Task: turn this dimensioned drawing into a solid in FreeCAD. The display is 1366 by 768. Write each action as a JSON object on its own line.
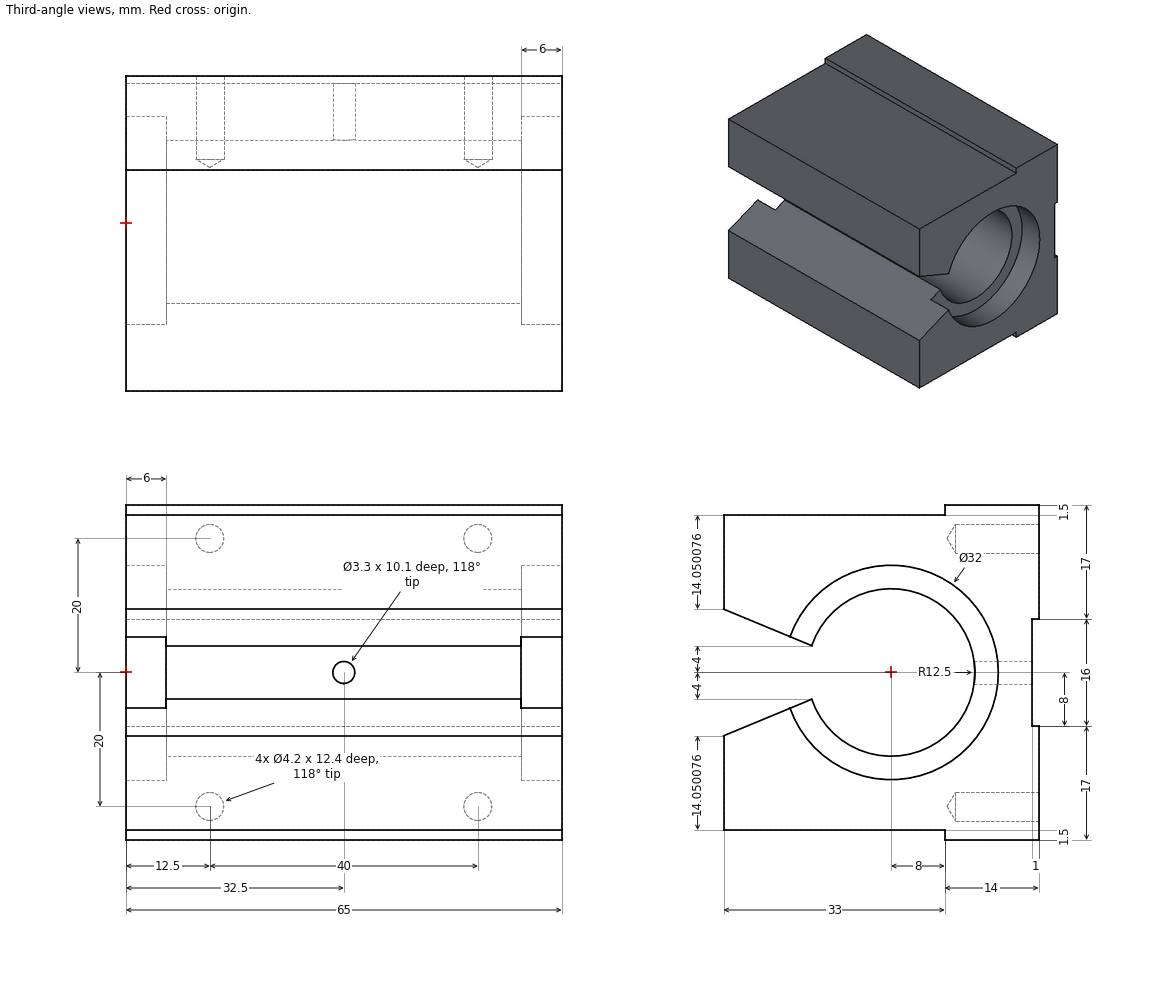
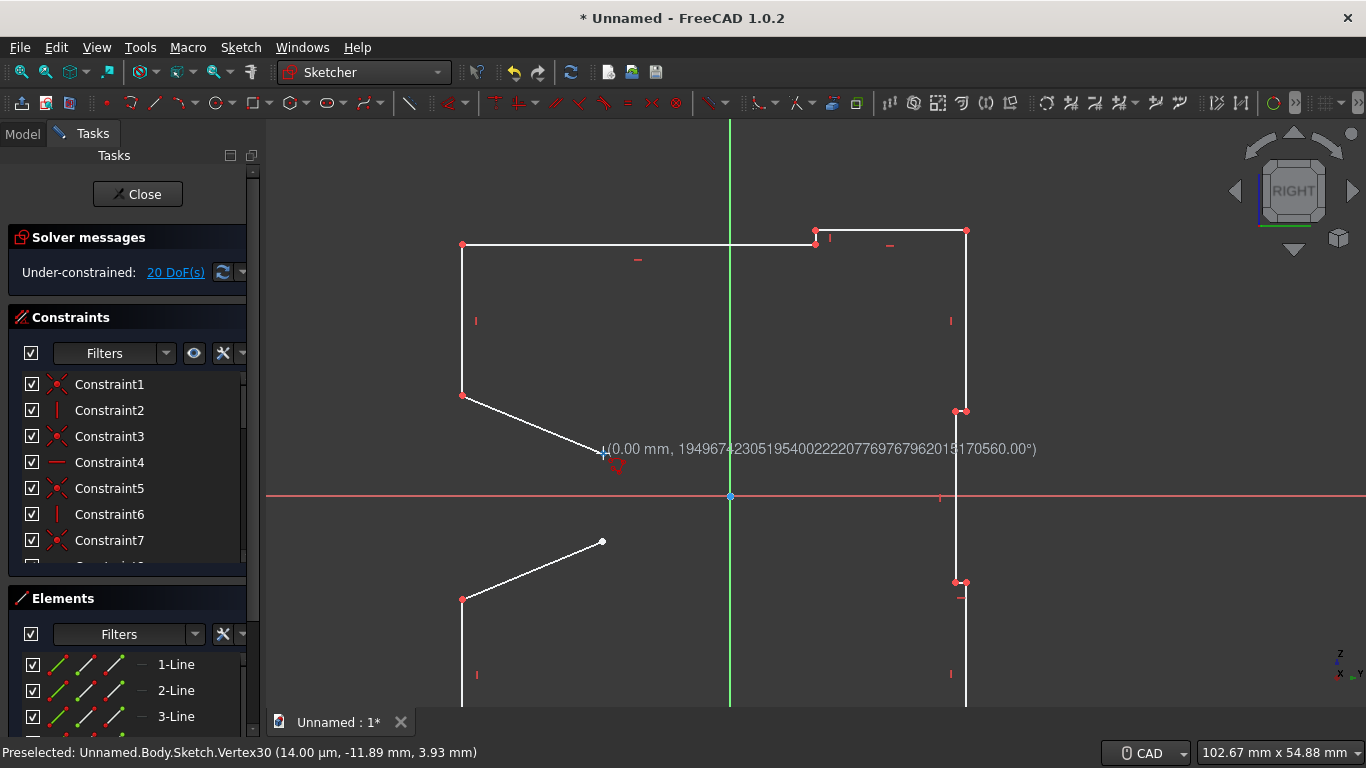
{"action": "key", "text": "g 3 a"}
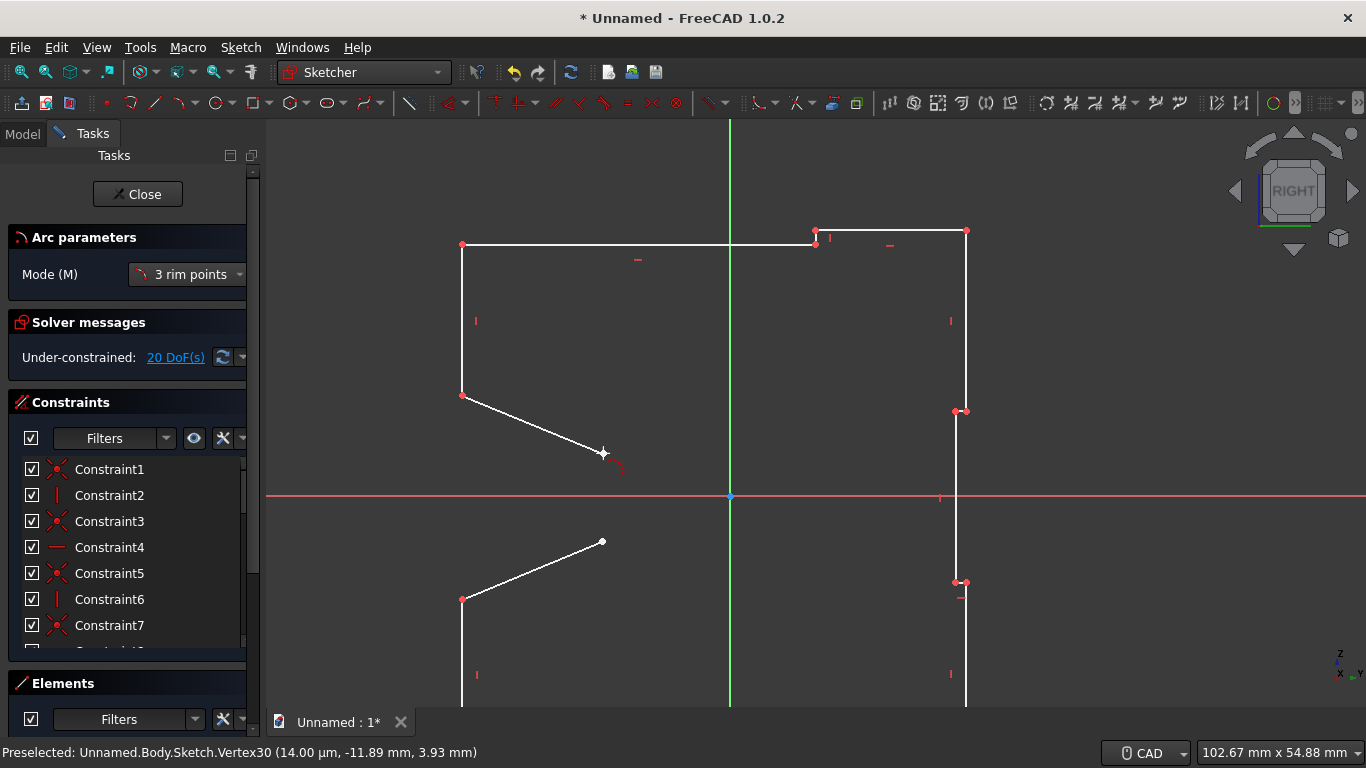
{"action": "left_click", "coordinate": [603, 454]}
{"action": "left_click", "coordinate": [603, 542]}
{"action": "left_click", "coordinate": [844, 568]}
{"action": "key", "text": "Escape"}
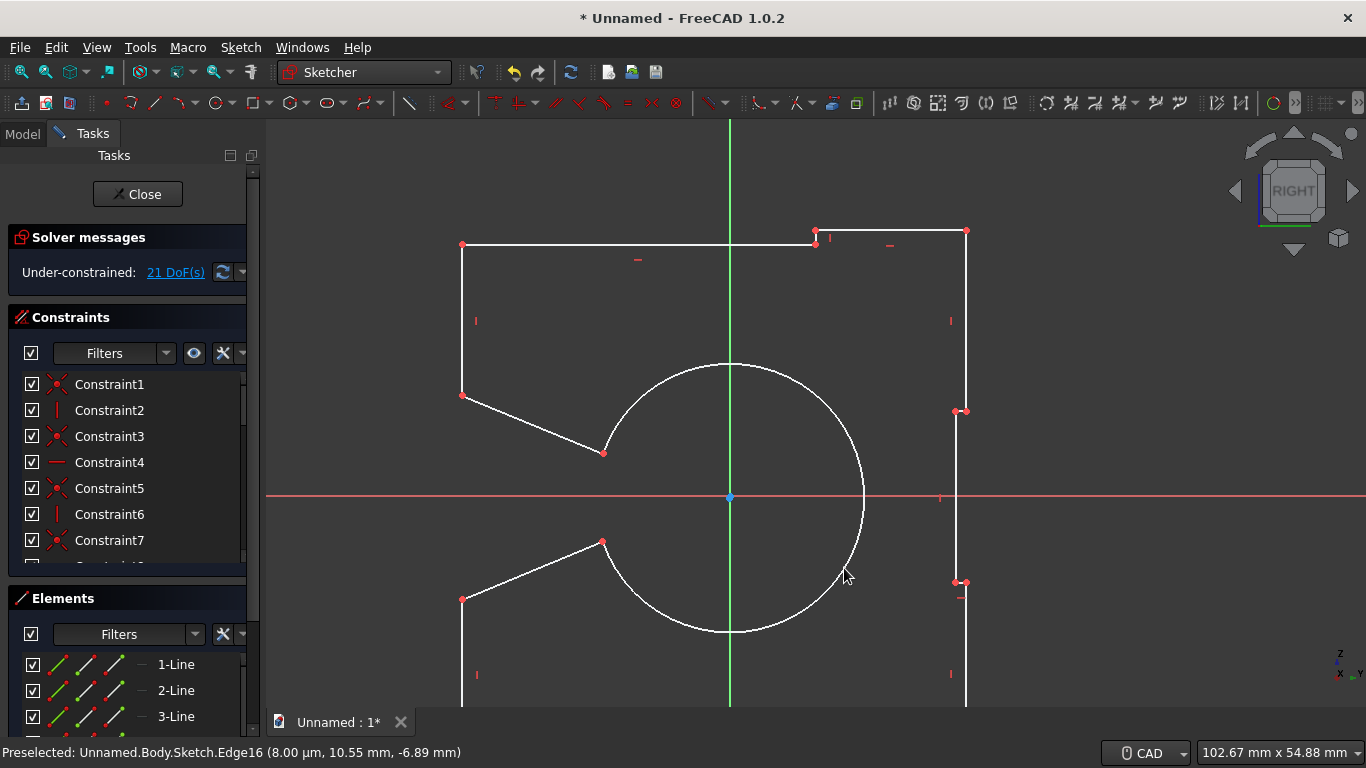
{"action": "scroll", "coordinate": [961, 411], "scroll_direction": "up", "scroll_amount": 5}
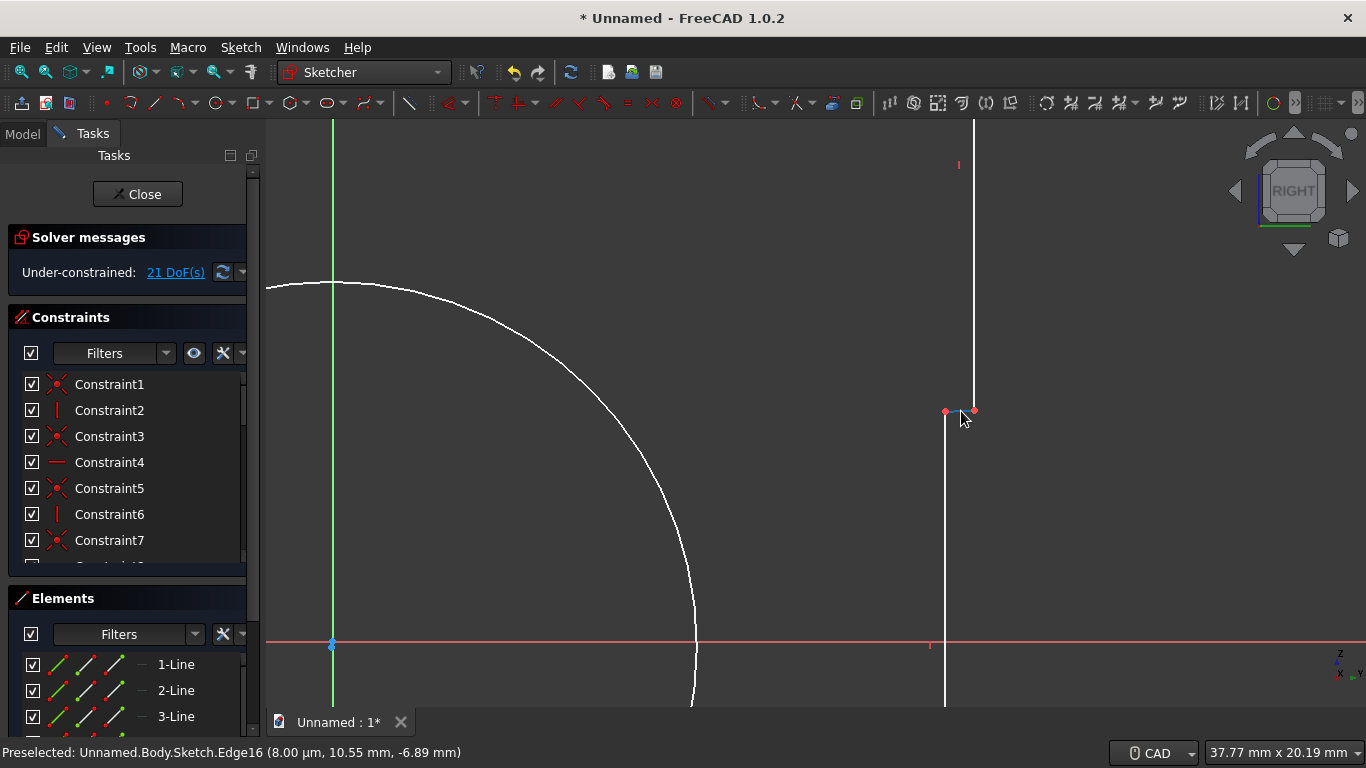
{"action": "left_click", "coordinate": [960, 411]}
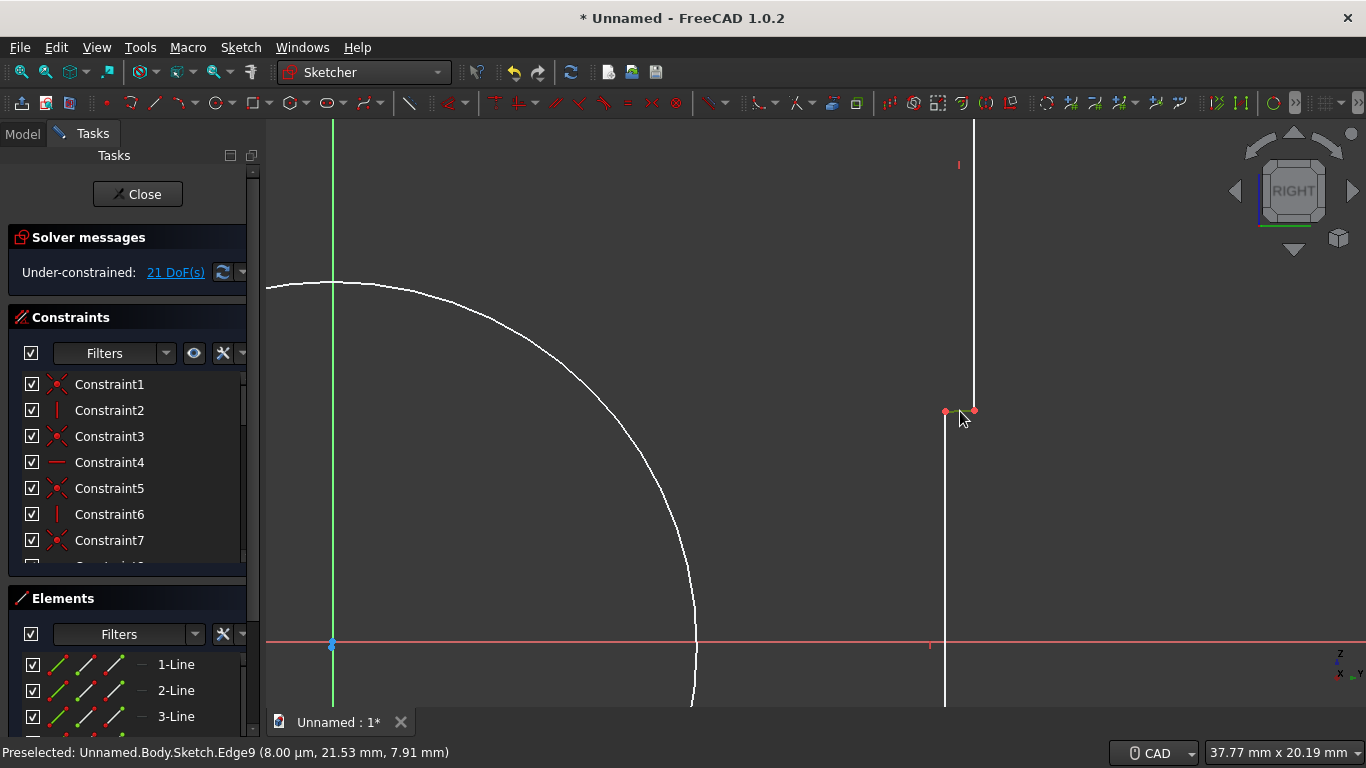
{"action": "key", "text": "h"}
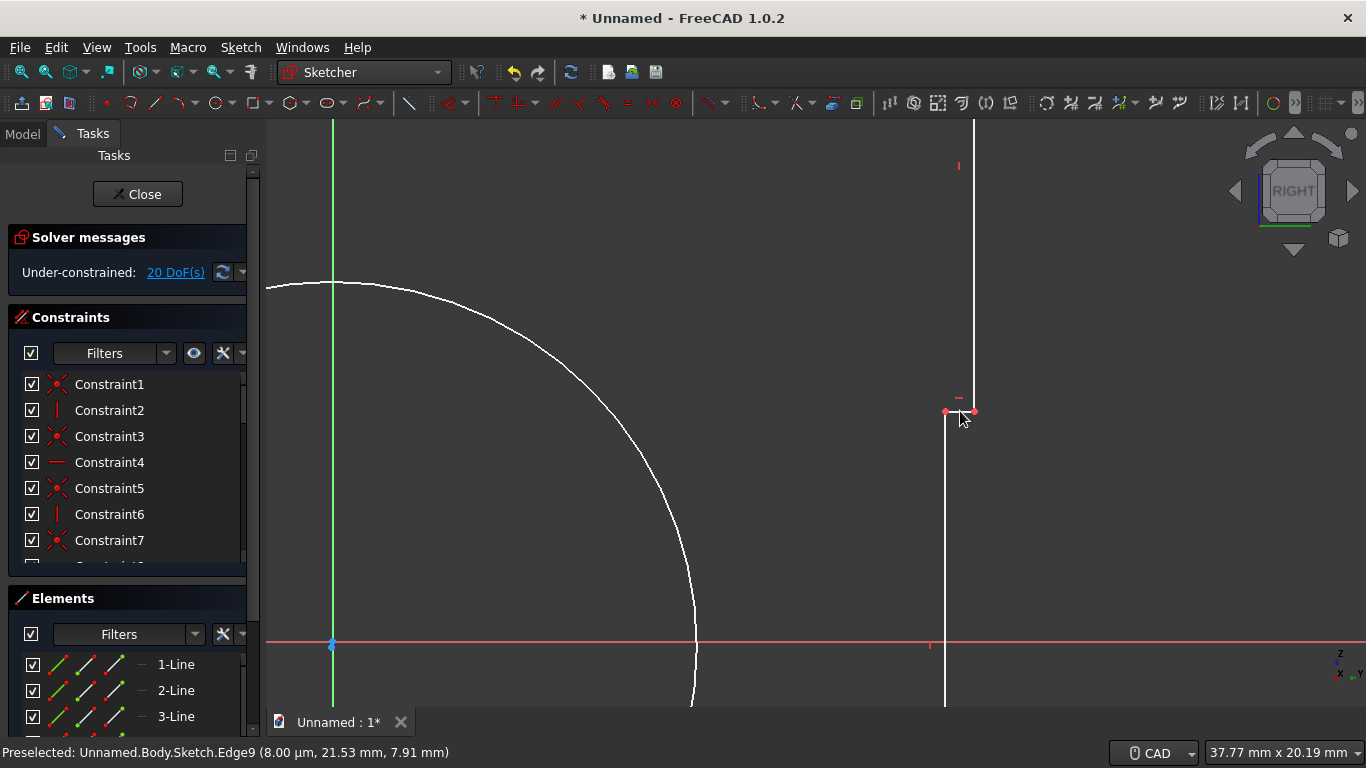
{"action": "scroll", "coordinate": [897, 338], "scroll_direction": "down", "scroll_amount": 7}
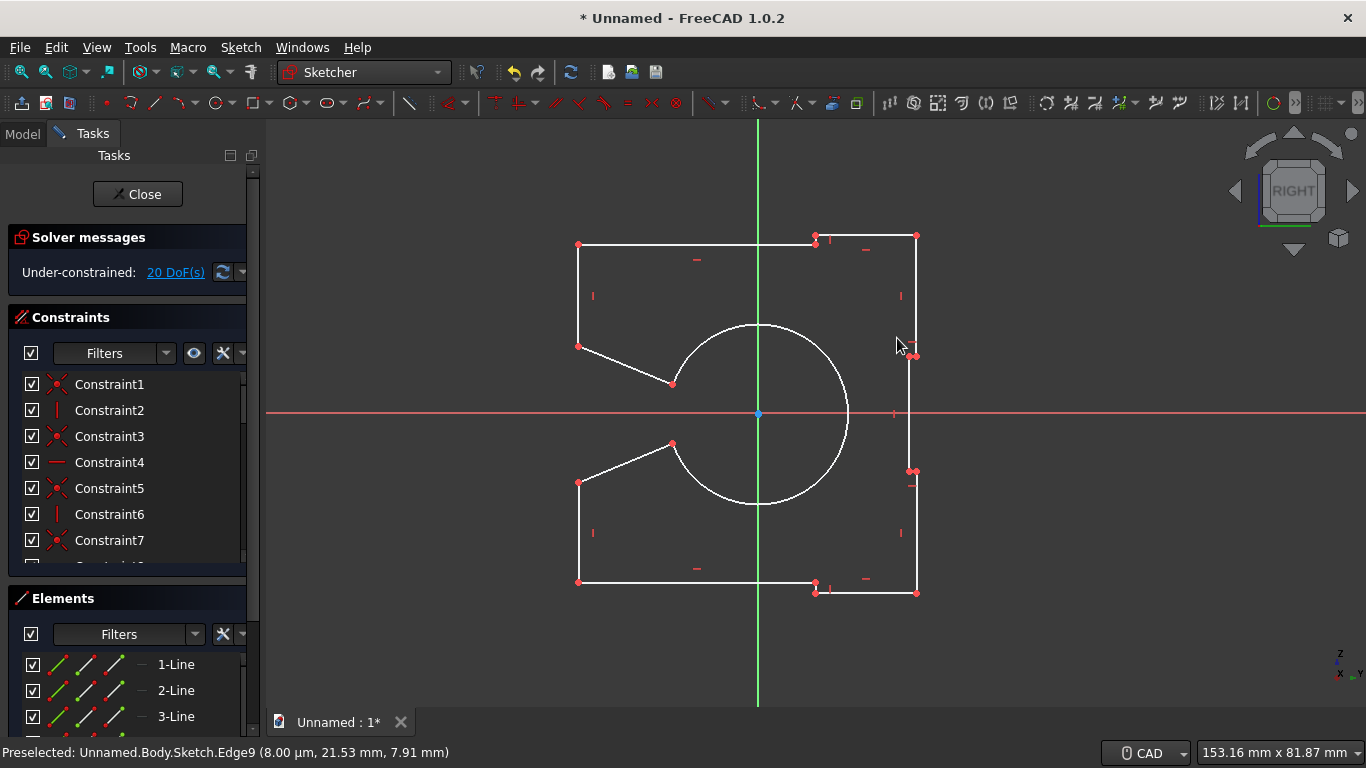
{"action": "left_click_drag", "start_coordinate": [748, 403], "coordinate": [768, 424]}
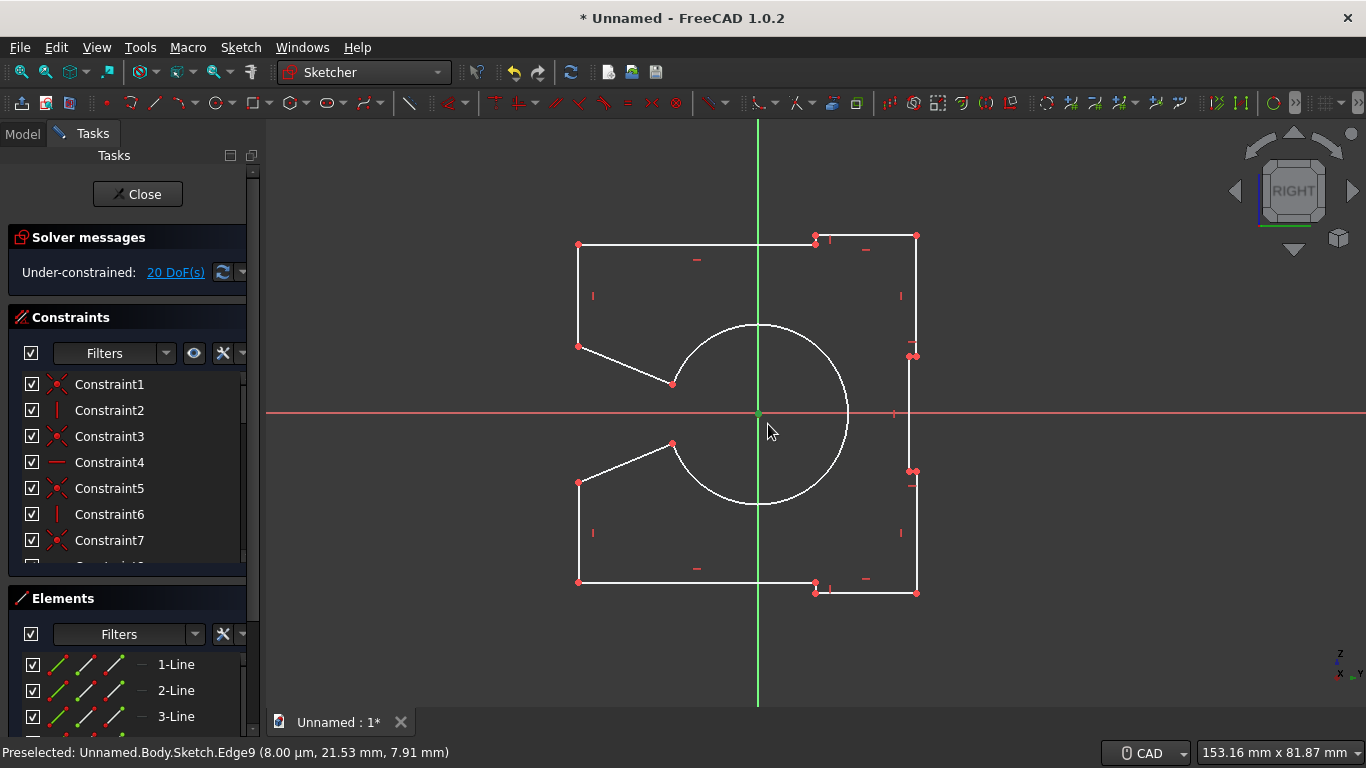
{"action": "left_click", "coordinate": [496, 104]}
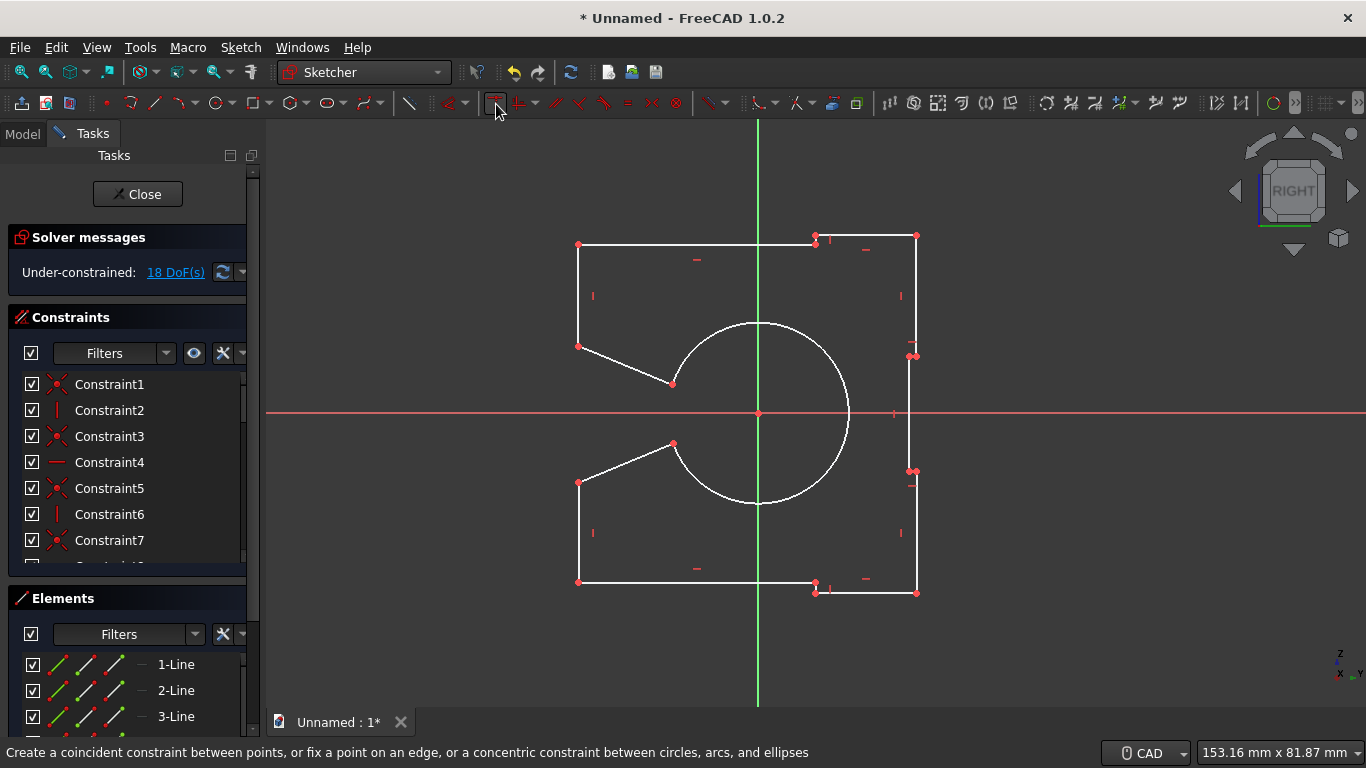
{"action": "left_click", "coordinate": [799, 494]}